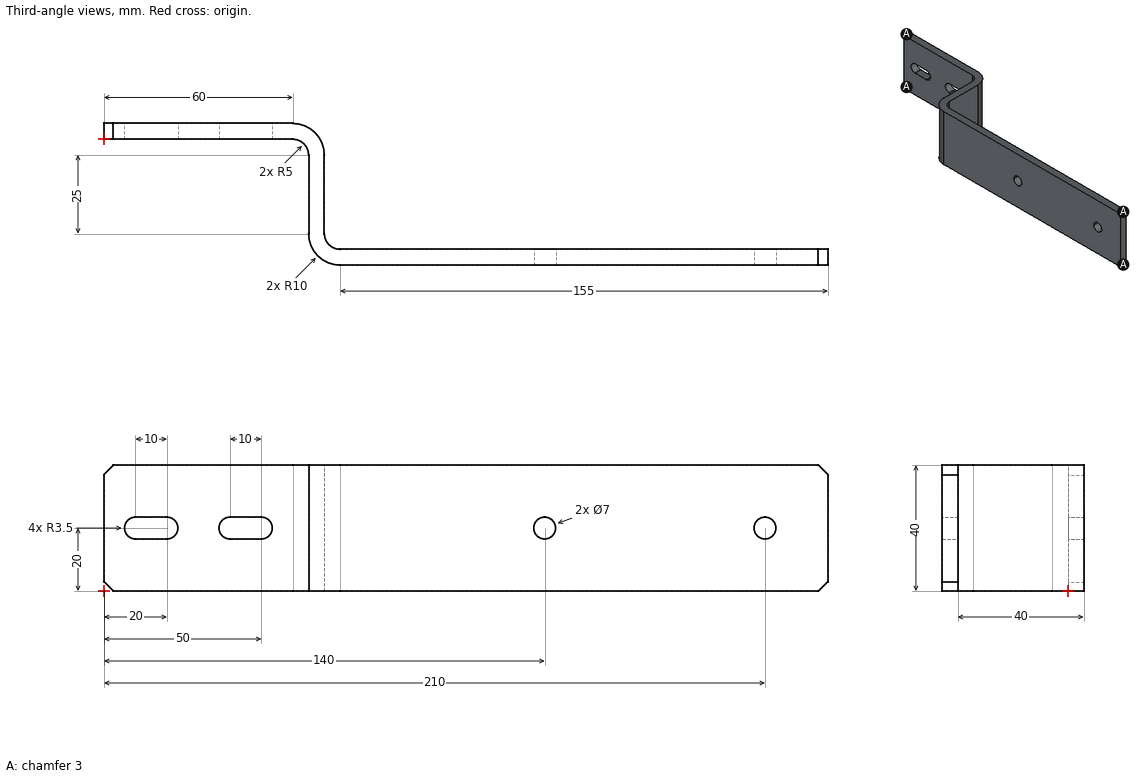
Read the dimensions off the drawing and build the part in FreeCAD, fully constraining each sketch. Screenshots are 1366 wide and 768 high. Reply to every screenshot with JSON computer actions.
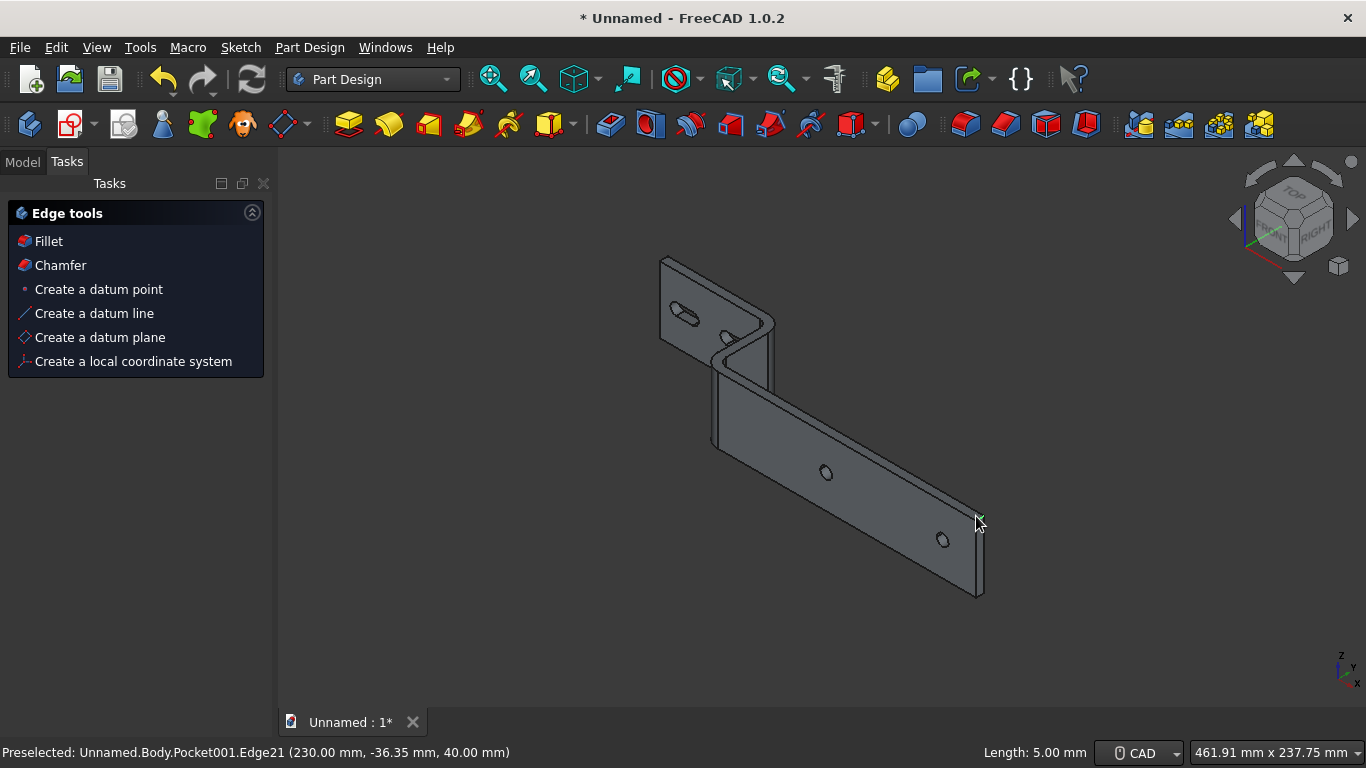
{"action": "scroll", "coordinate": [664, 335], "scroll_direction": "up", "scroll_amount": 7}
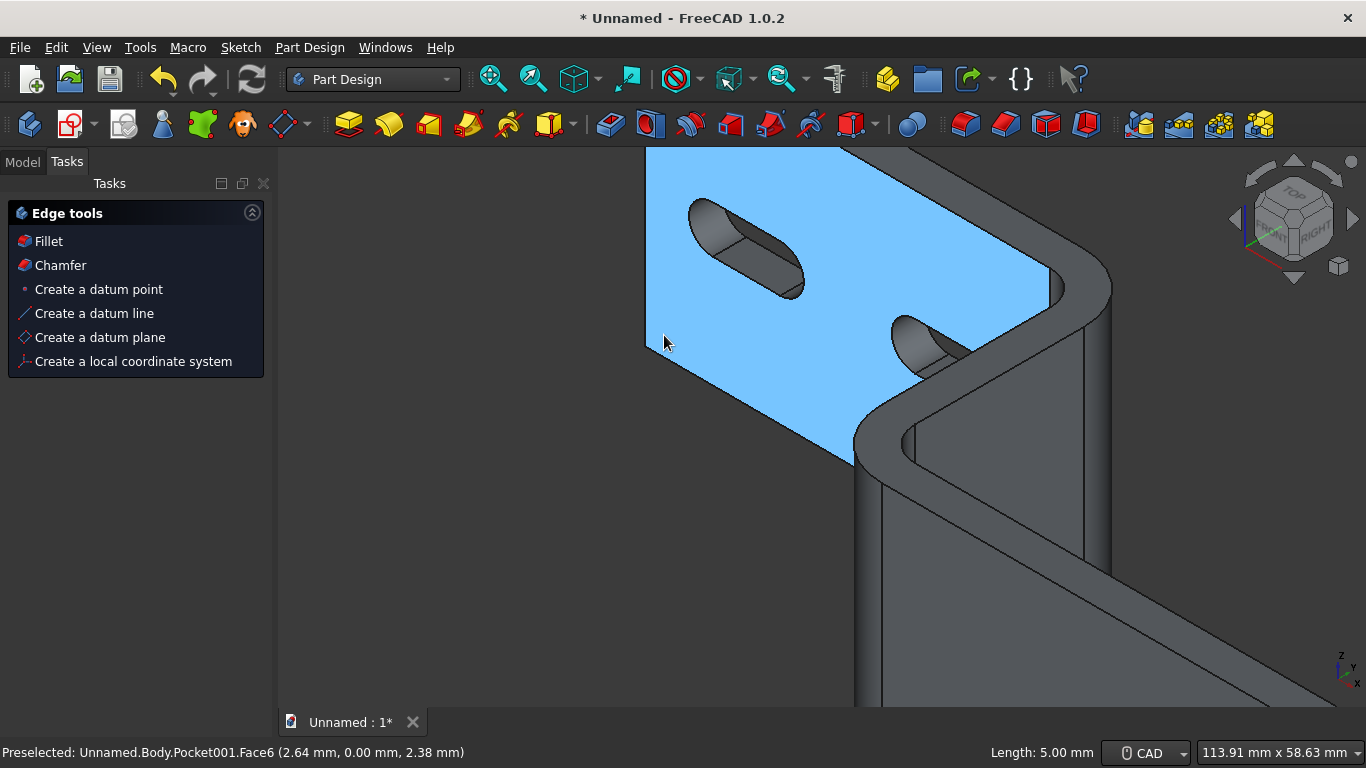
{"action": "left_click", "coordinate": [494, 80]}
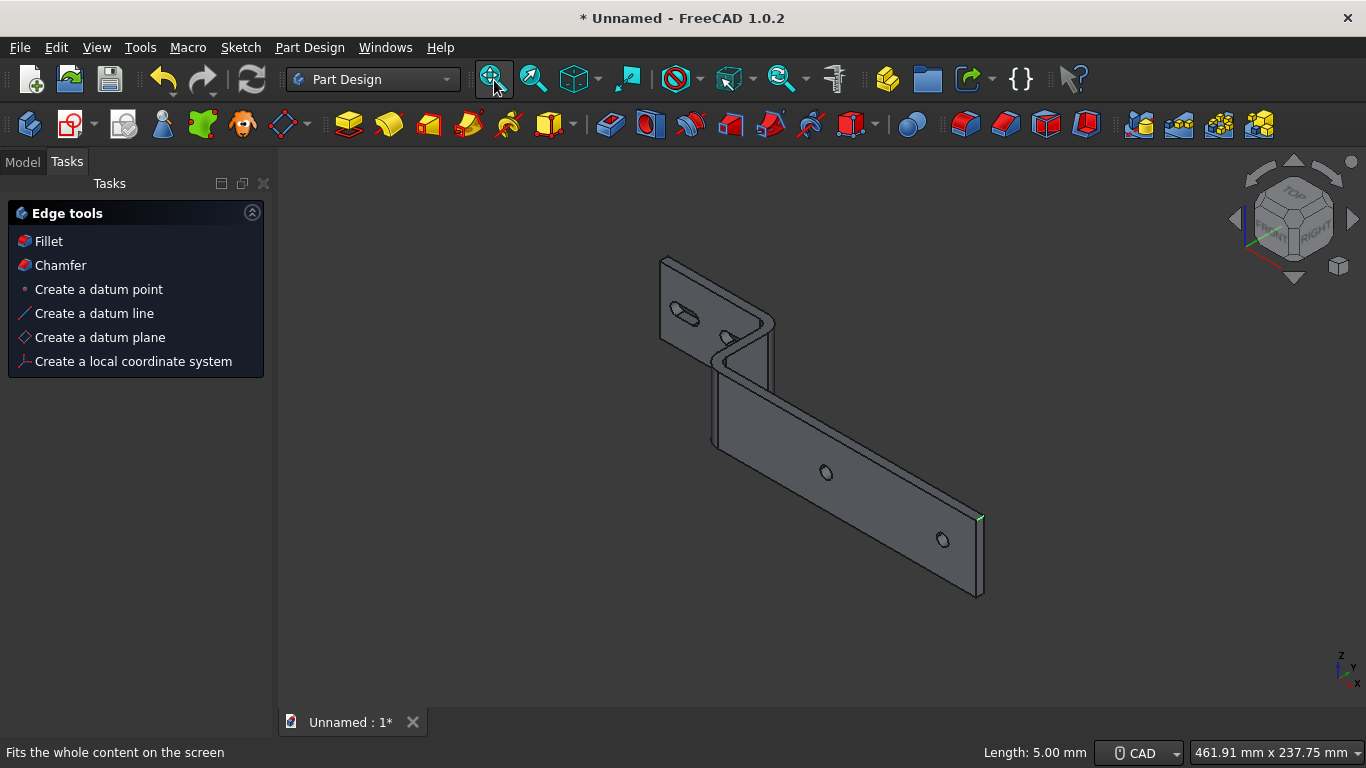
{"action": "key", "text": "2"}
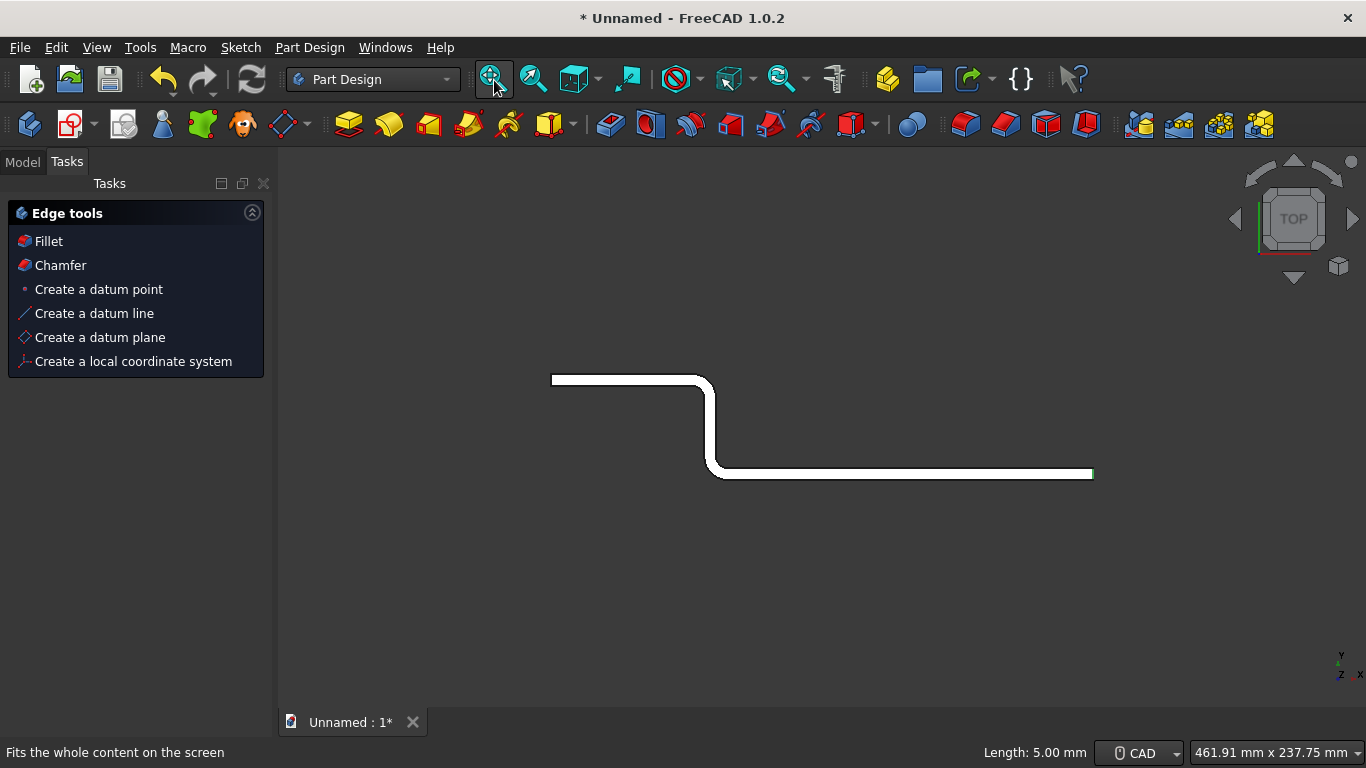
{"action": "scroll", "coordinate": [551, 379], "scroll_direction": "up", "scroll_amount": 7}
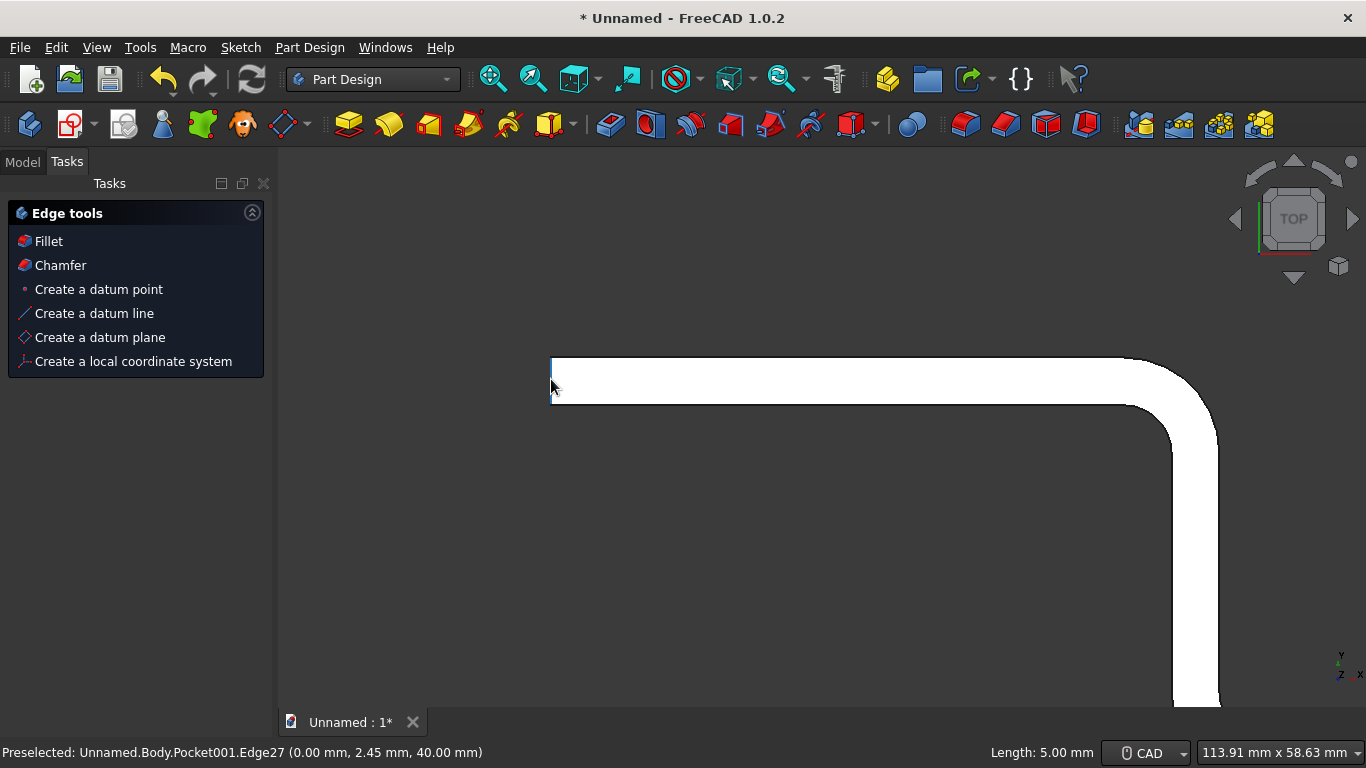
{"action": "left_click", "coordinate": [551, 380], "text": "ctrl"}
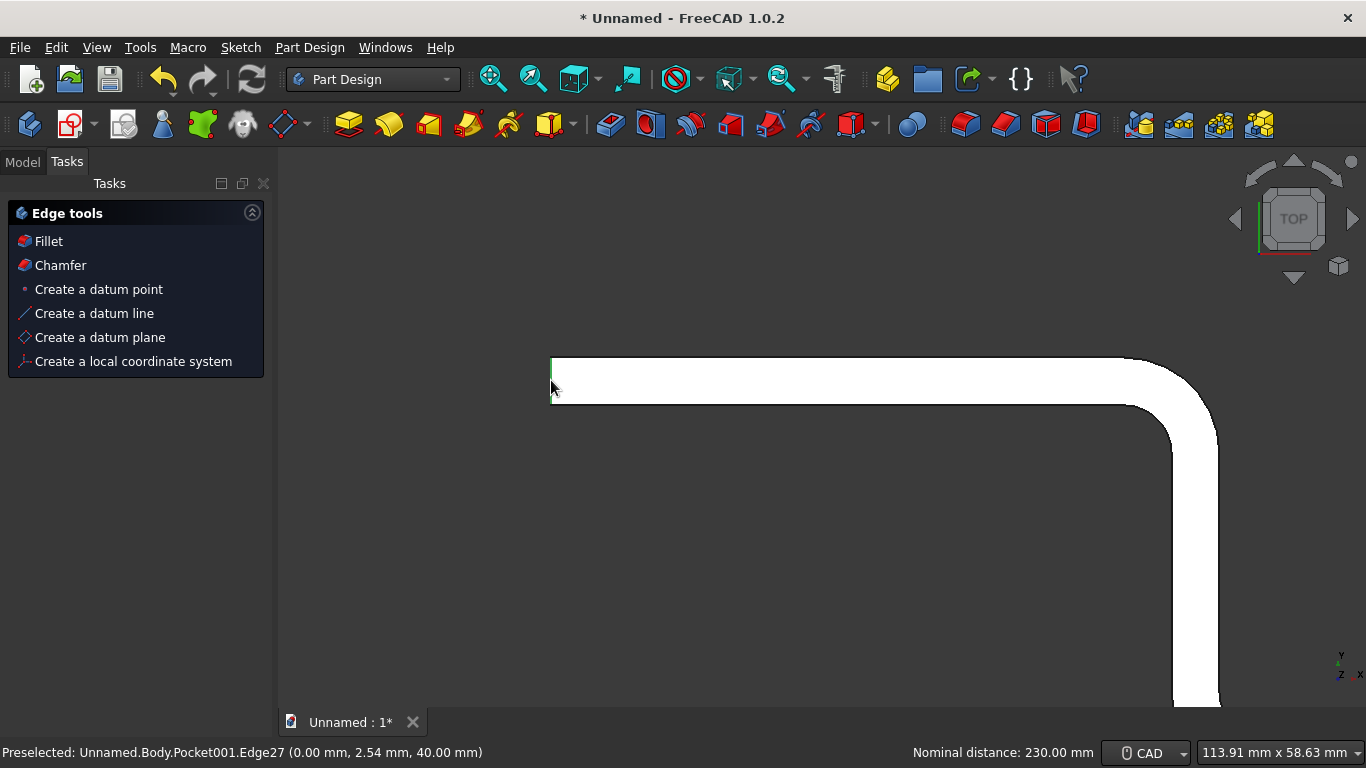
{"action": "left_click", "coordinate": [494, 80]}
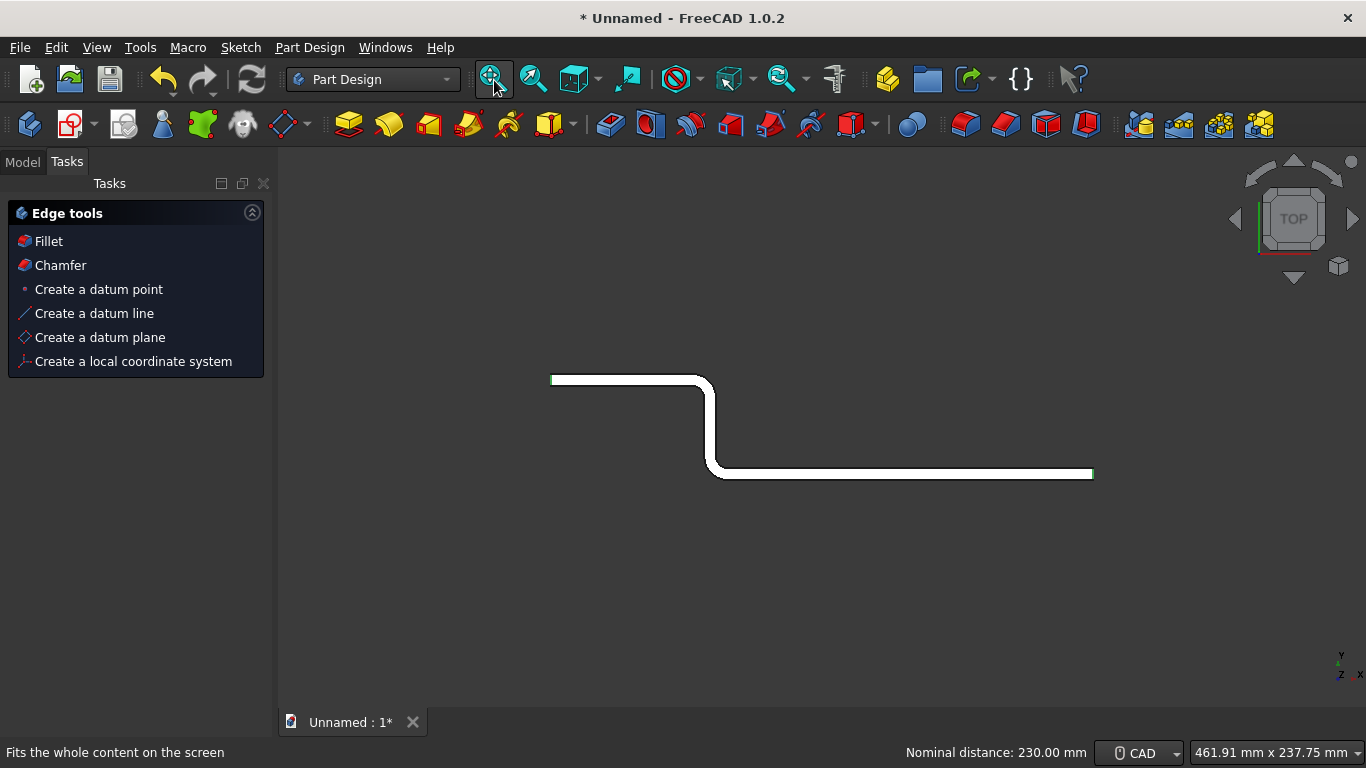
{"action": "key", "text": "1"}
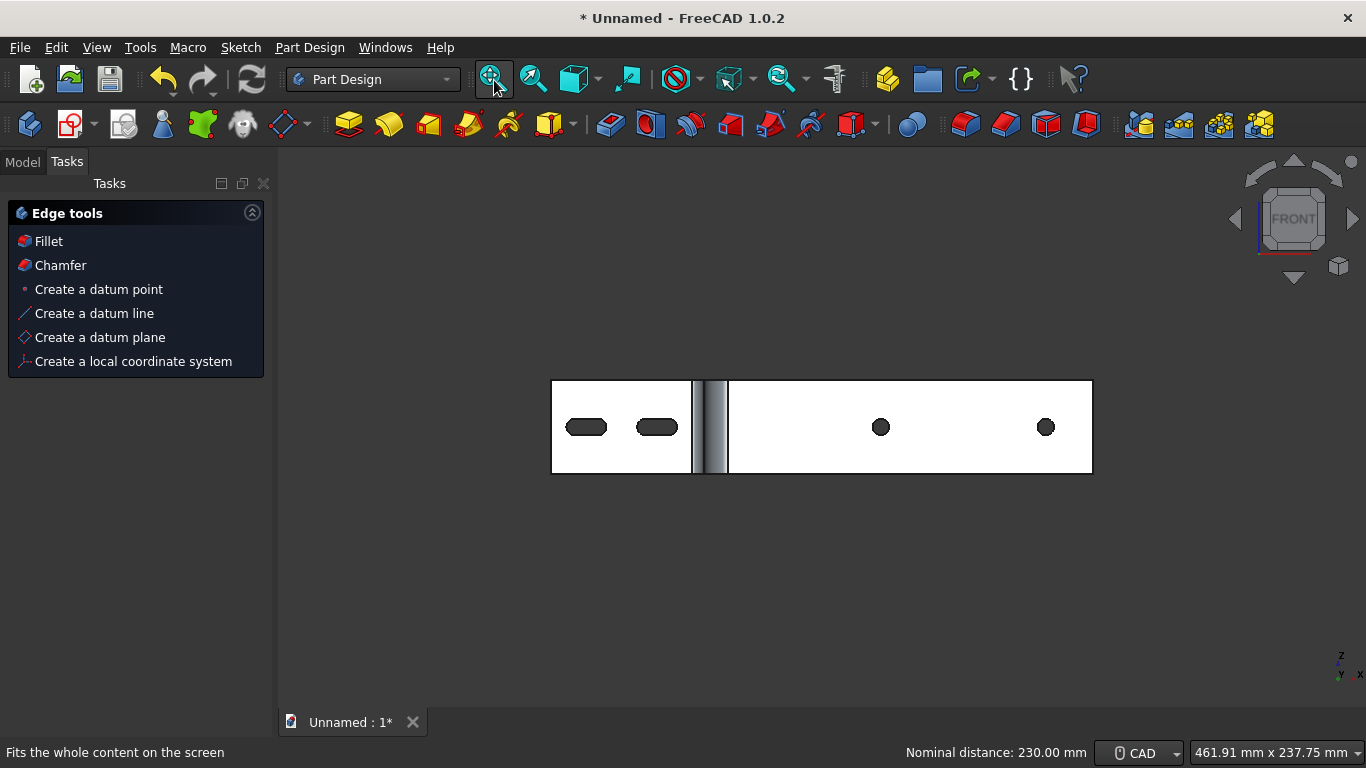
{"action": "scroll", "coordinate": [551, 473], "scroll_direction": "up", "scroll_amount": 7}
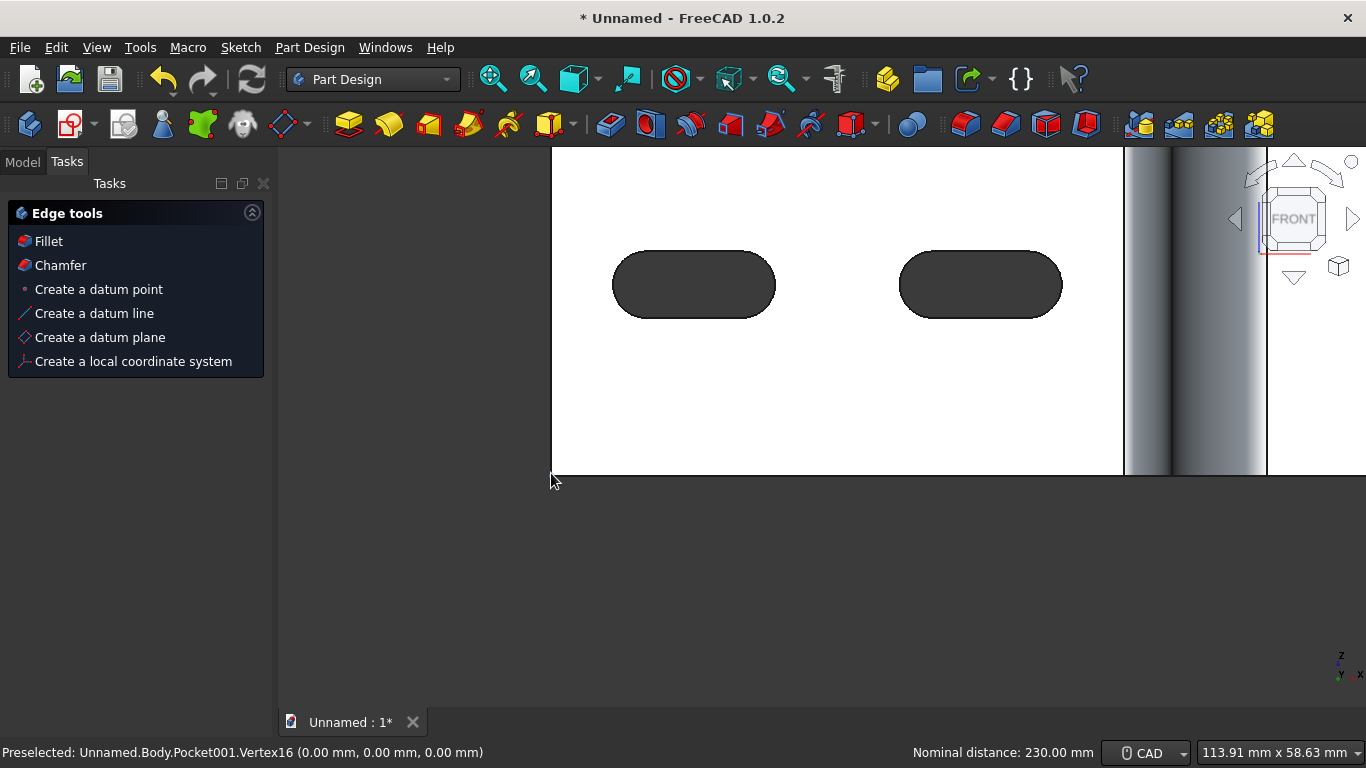
{"action": "left_click", "coordinate": [494, 80]}